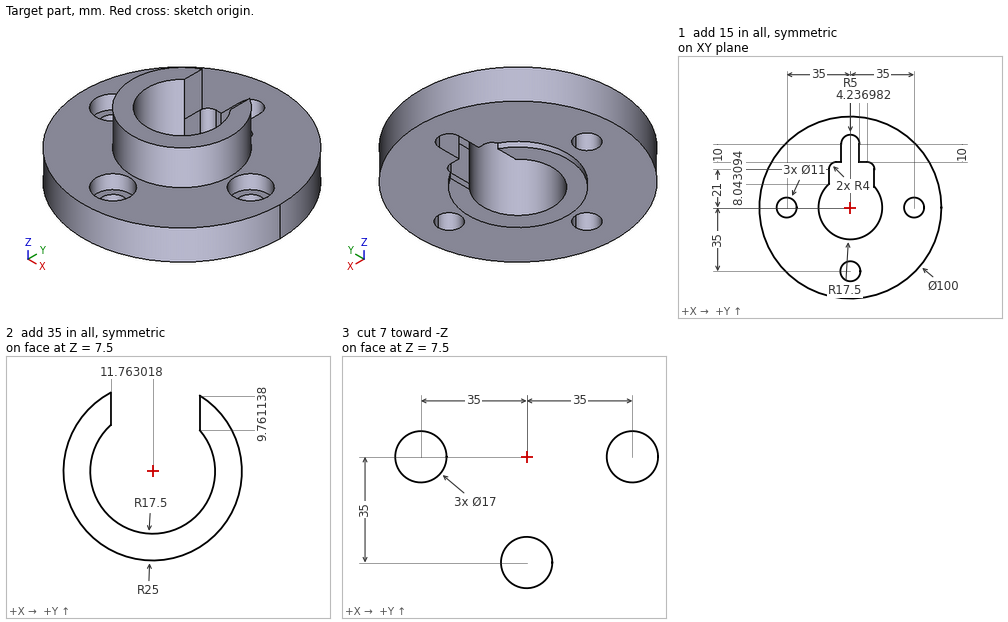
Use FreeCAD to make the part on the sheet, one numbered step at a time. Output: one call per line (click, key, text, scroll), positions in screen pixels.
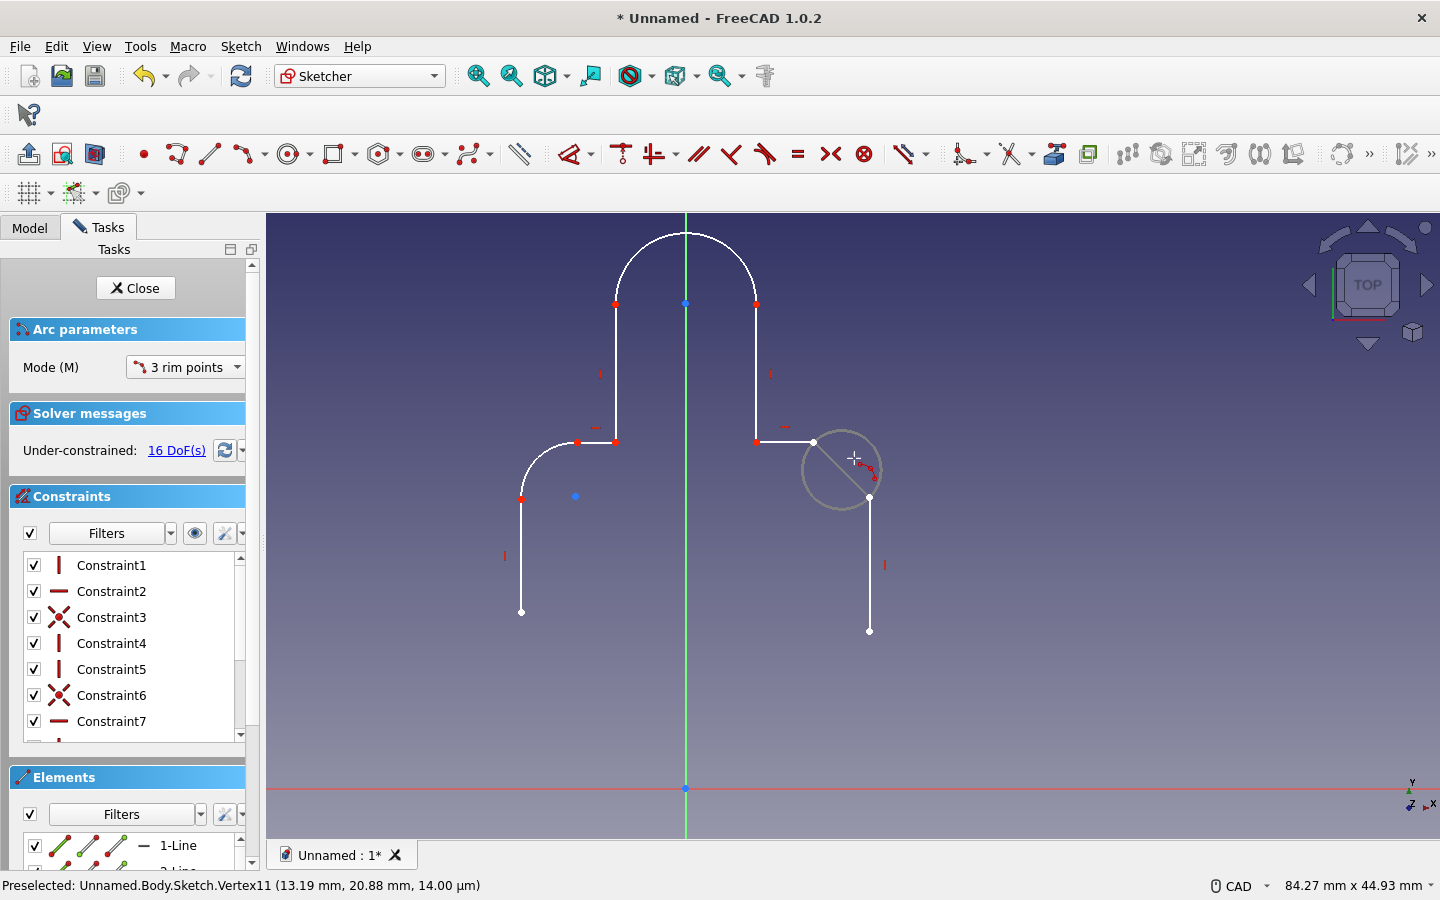
click(854, 457)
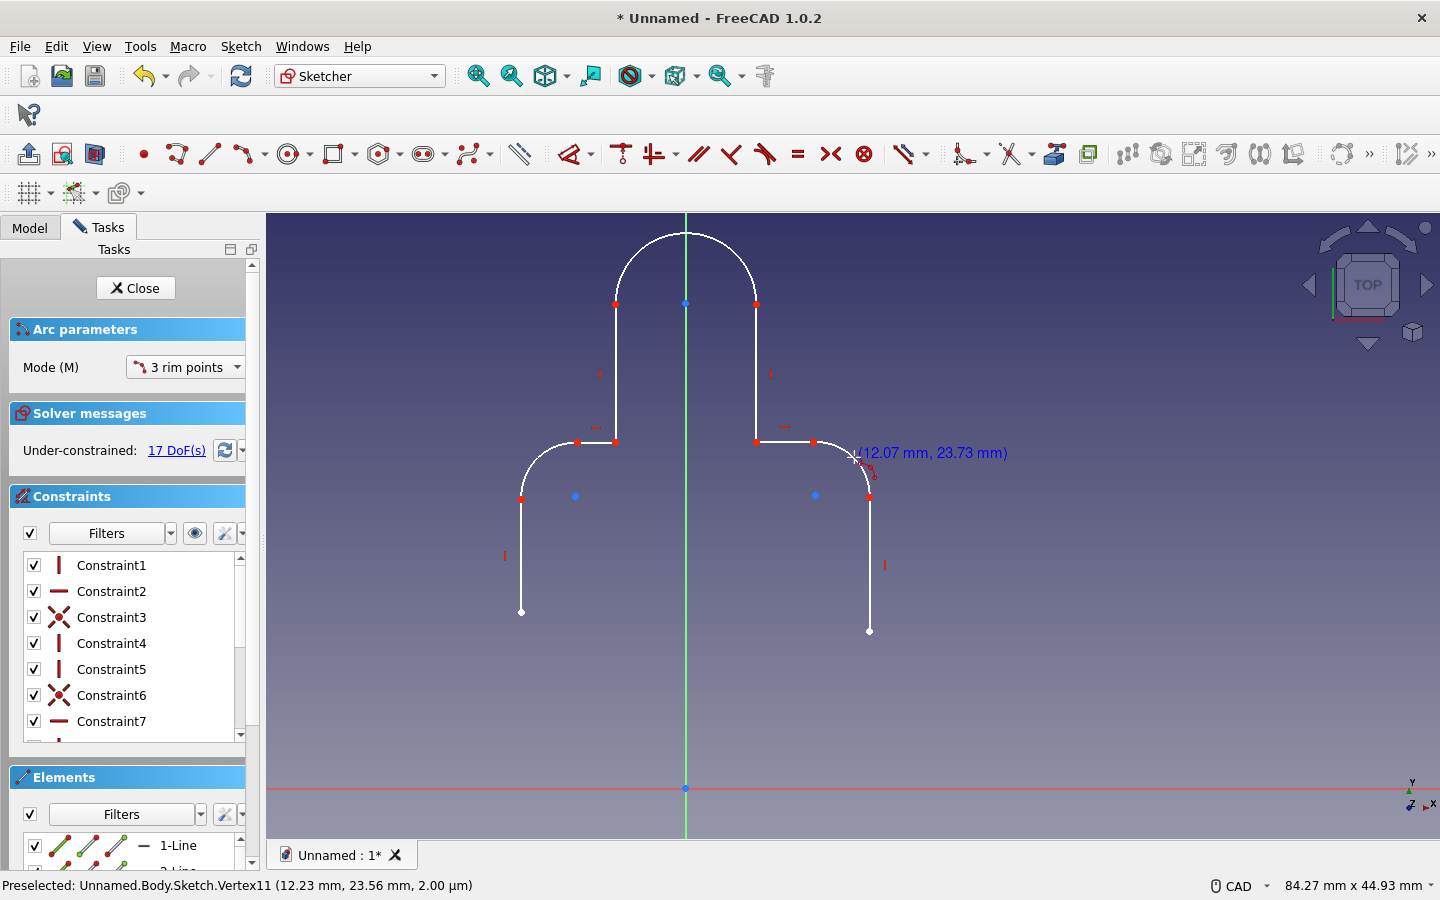
click(870, 631)
click(521, 612)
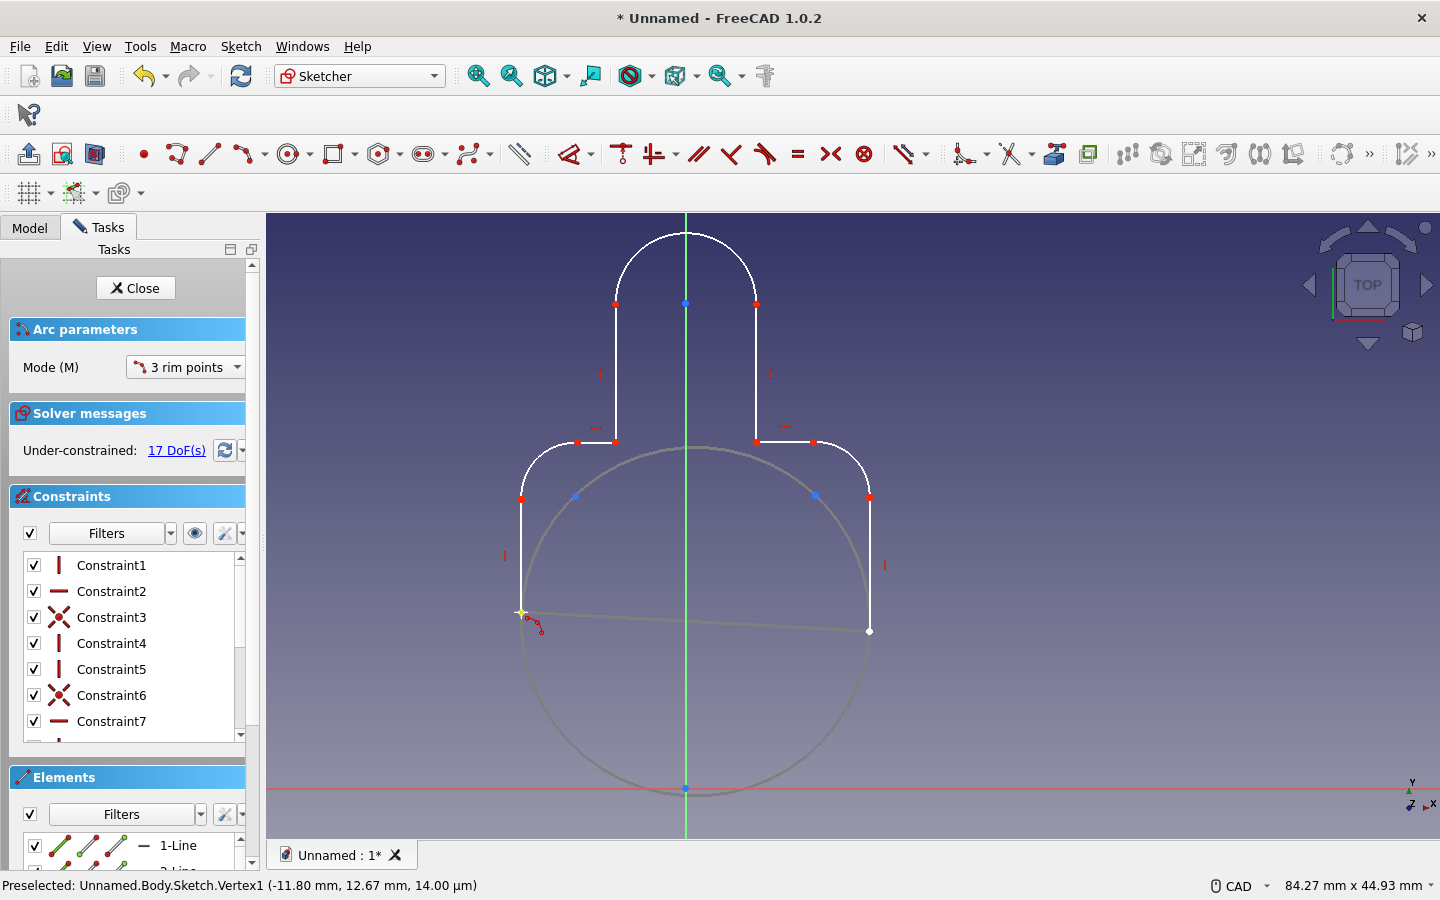
scroll(827, 413, down, 6)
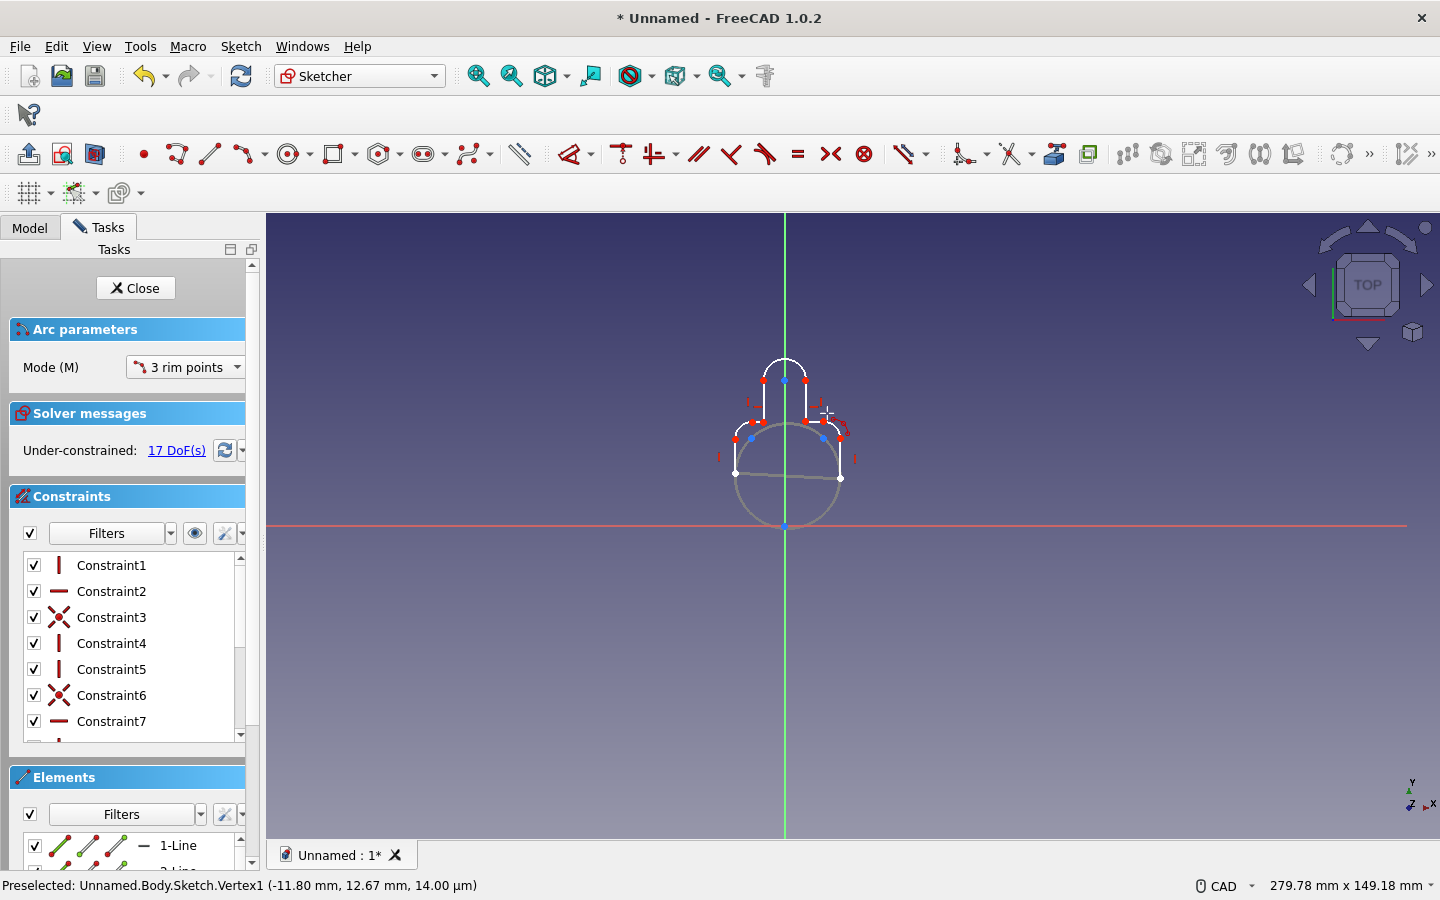
click(748, 590)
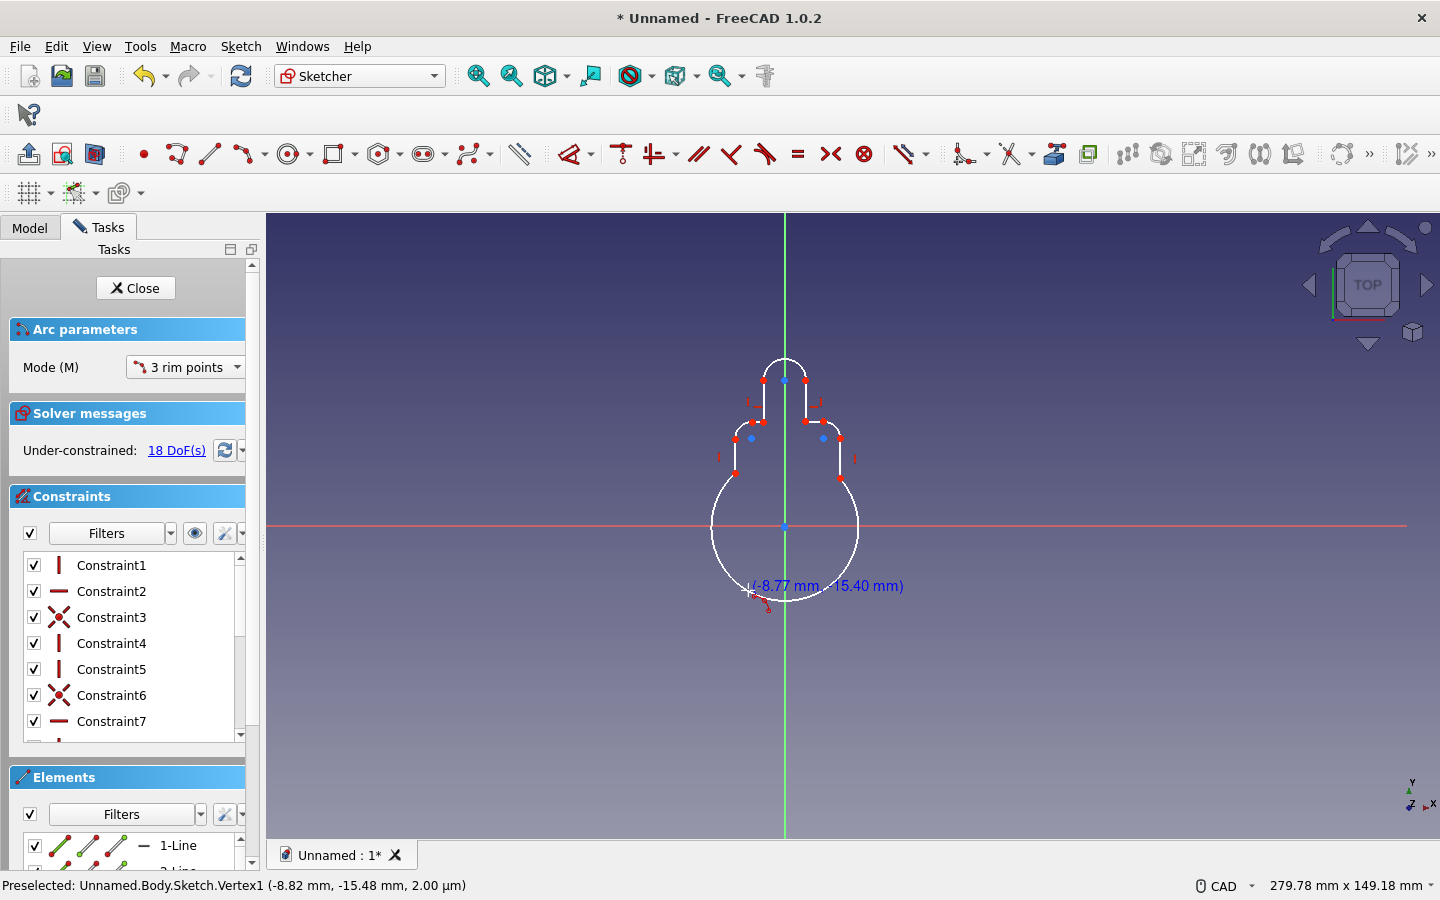
click(288, 154)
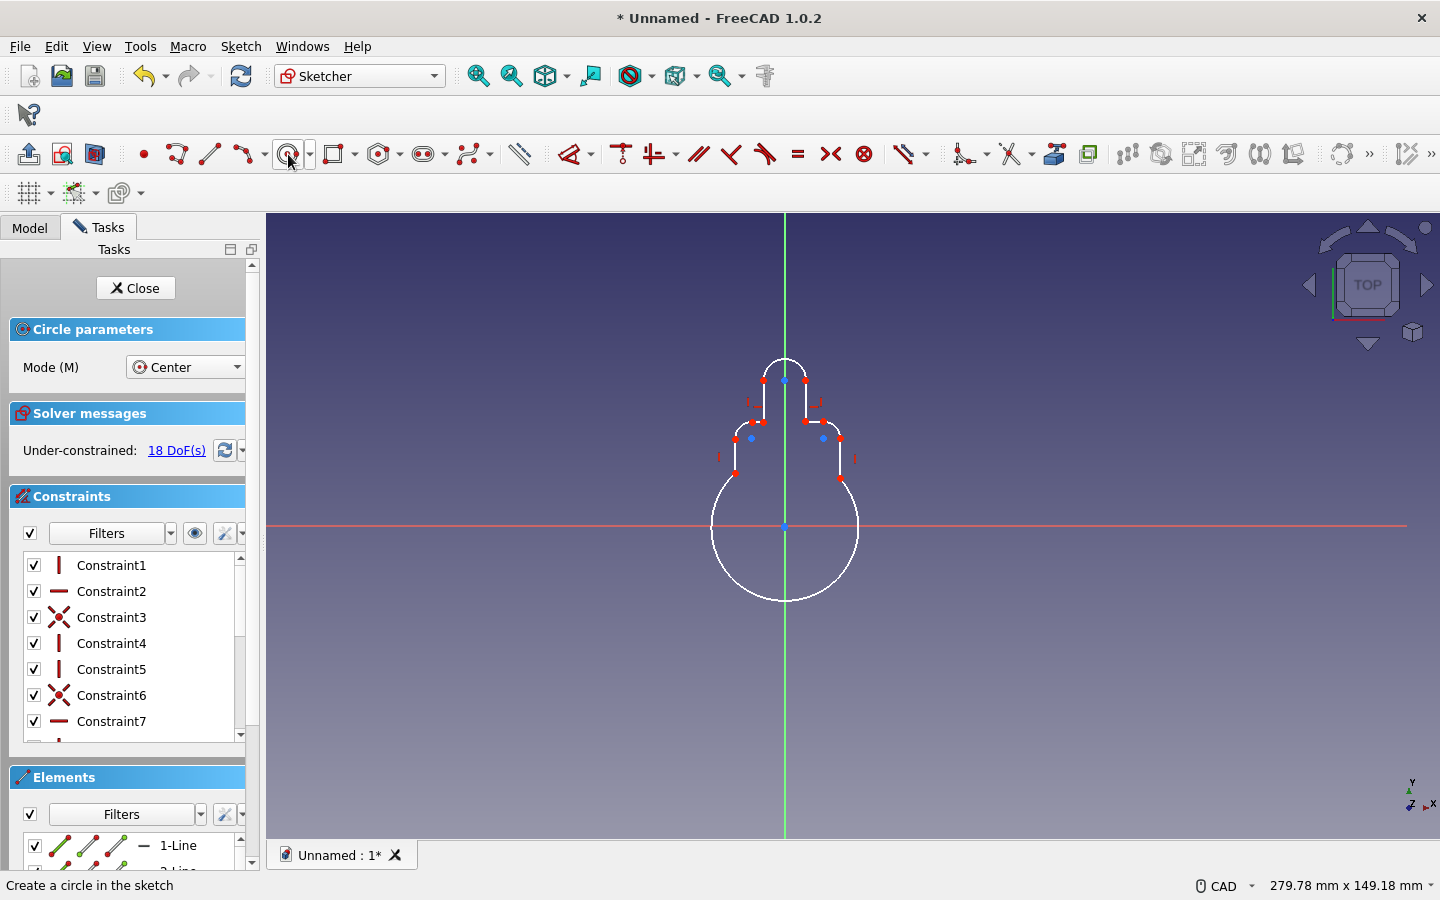
click(785, 526)
click(933, 378)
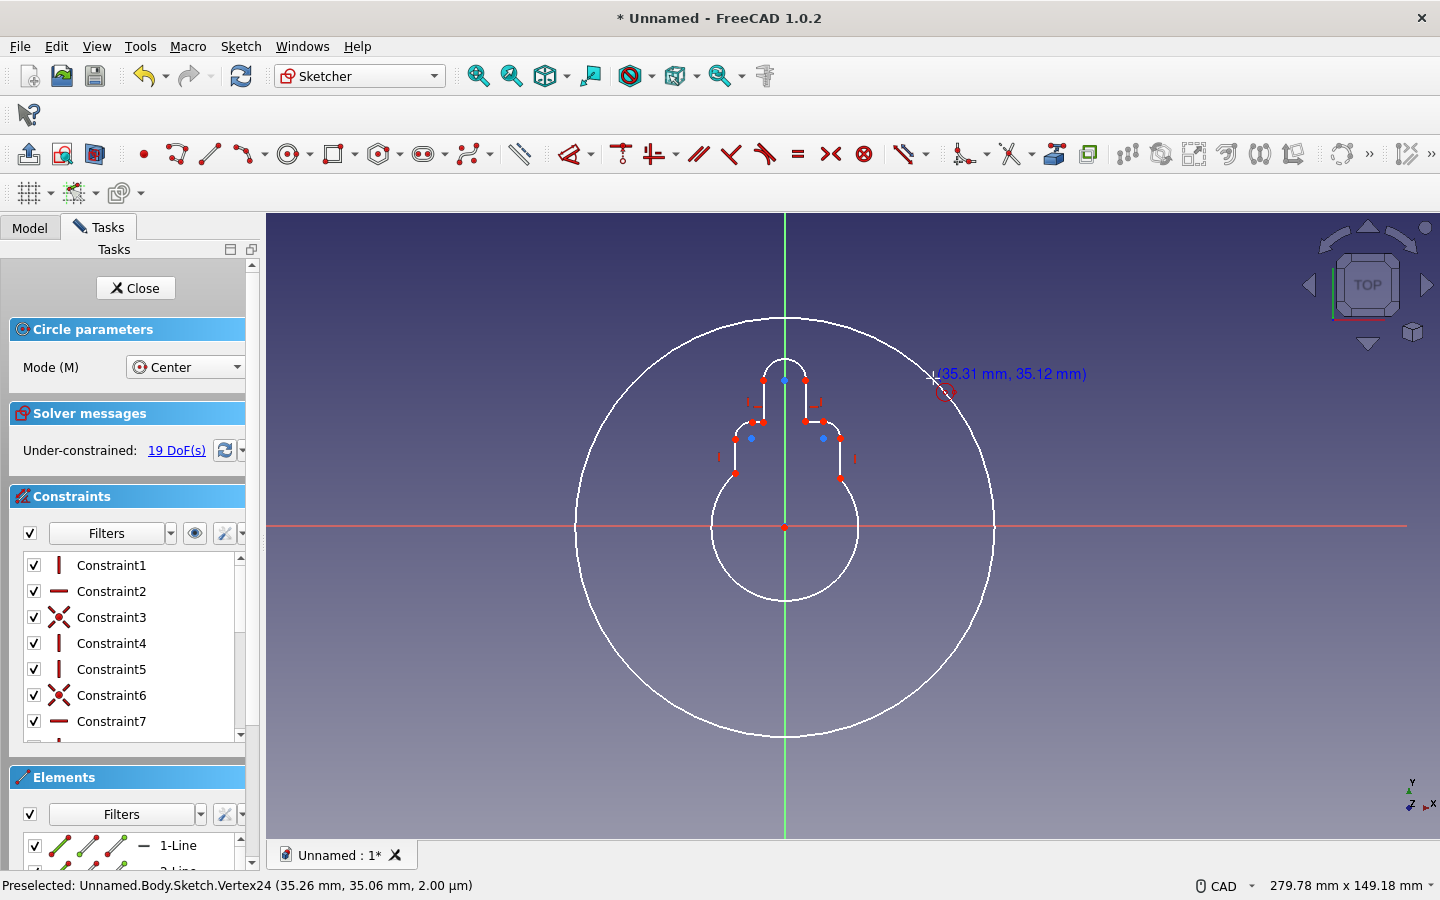
click(785, 673)
click(801, 657)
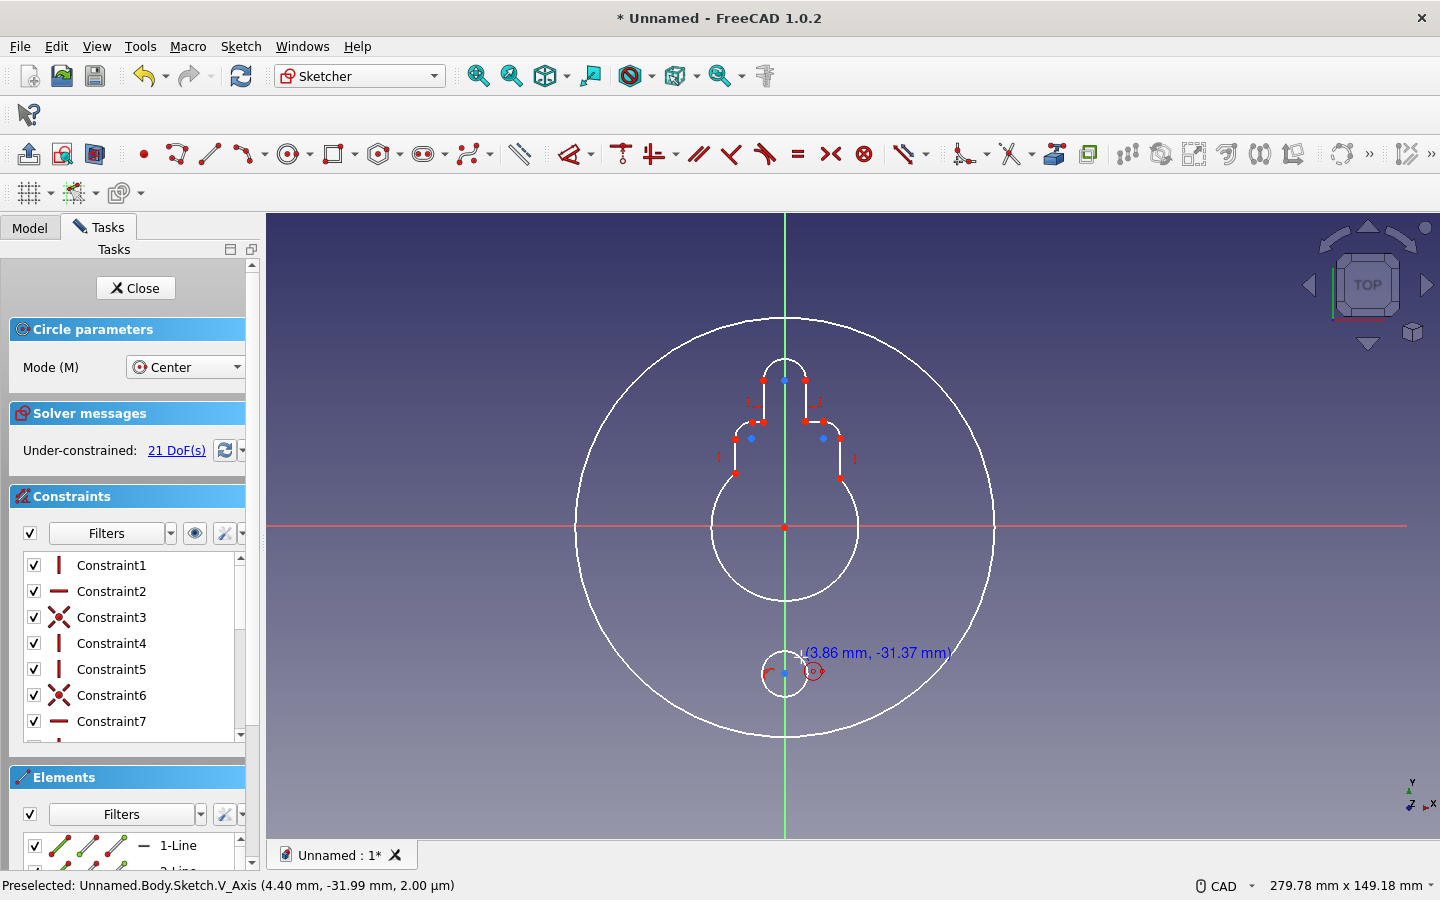
click(638, 526)
click(654, 510)